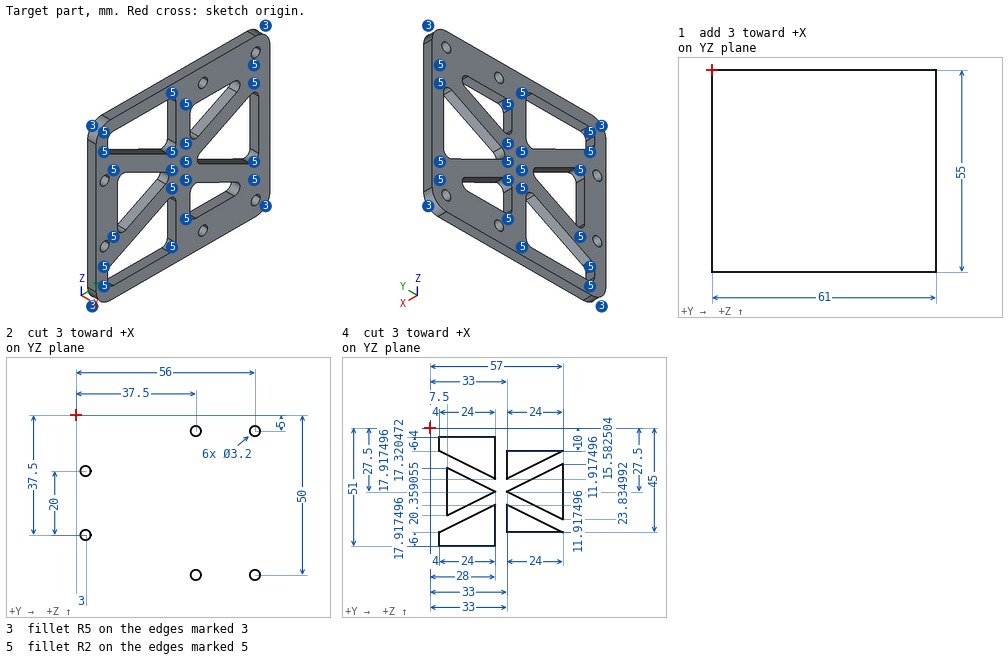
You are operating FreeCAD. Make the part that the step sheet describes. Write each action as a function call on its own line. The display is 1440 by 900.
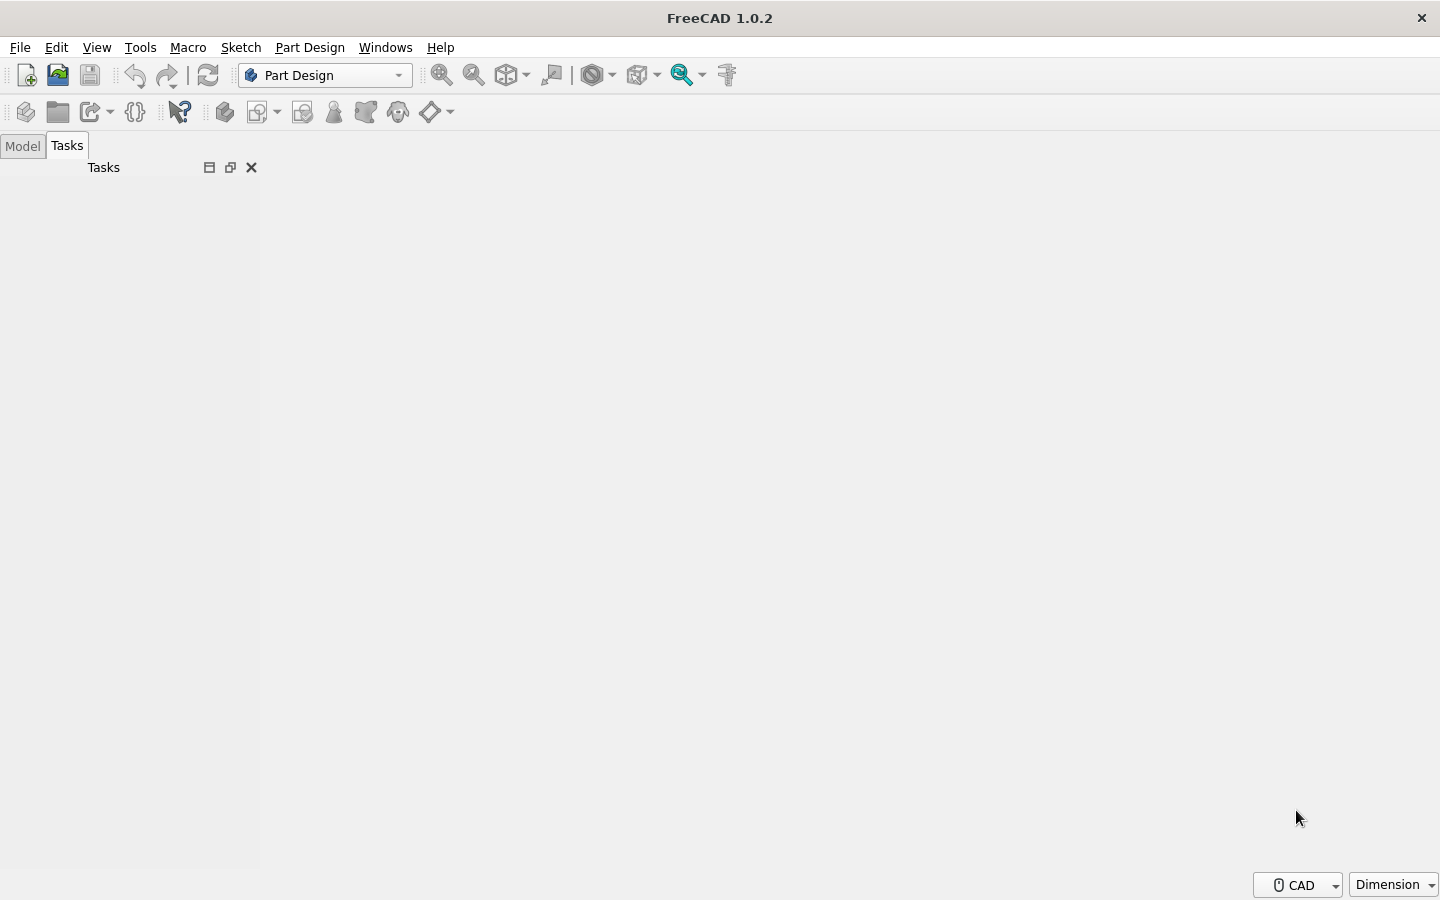
key(ctrl+n)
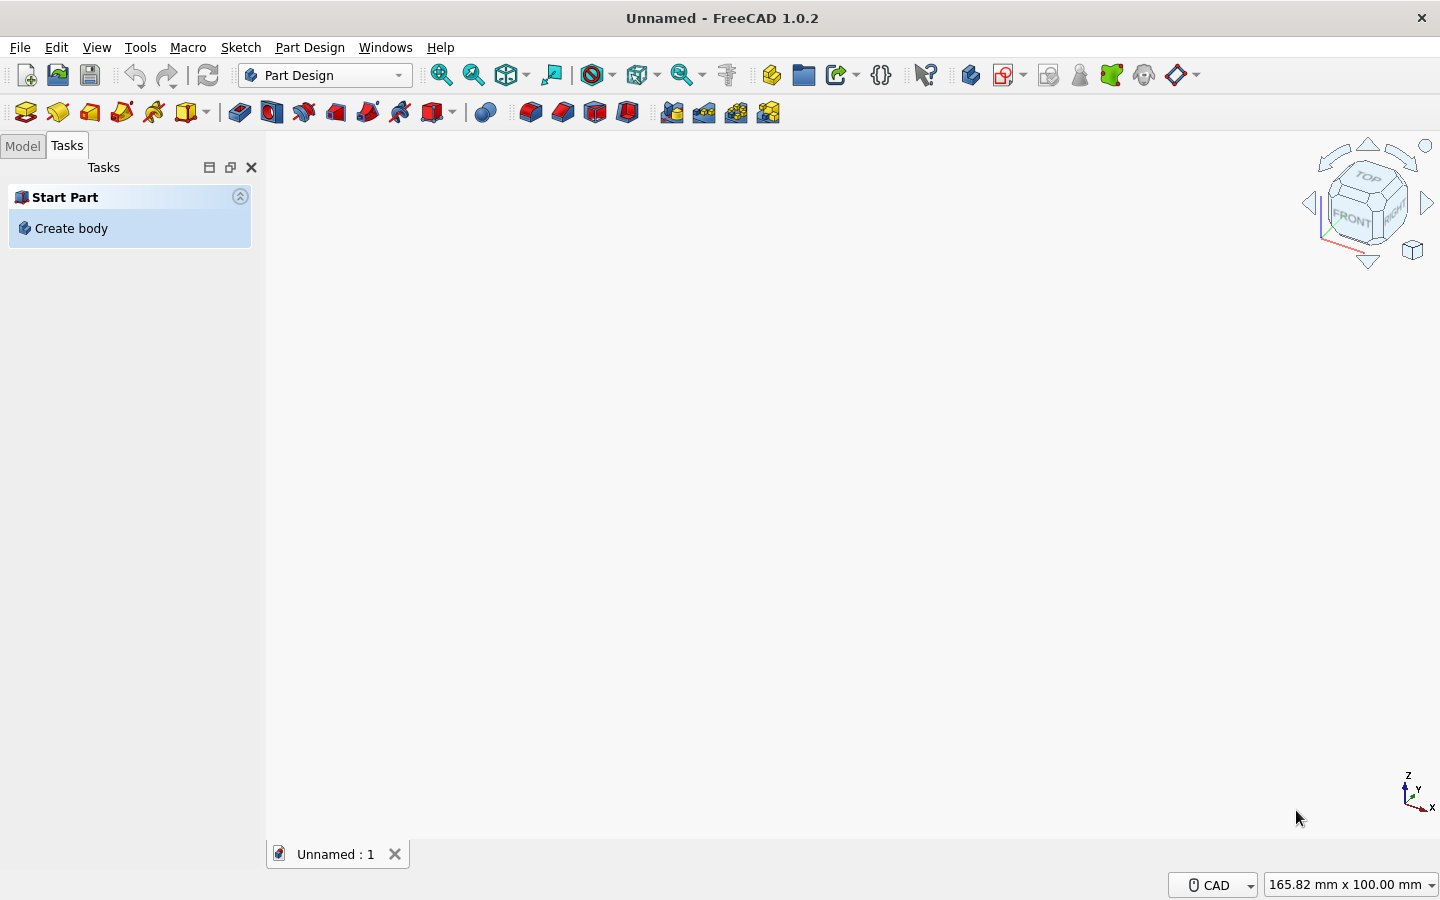
click(1004, 76)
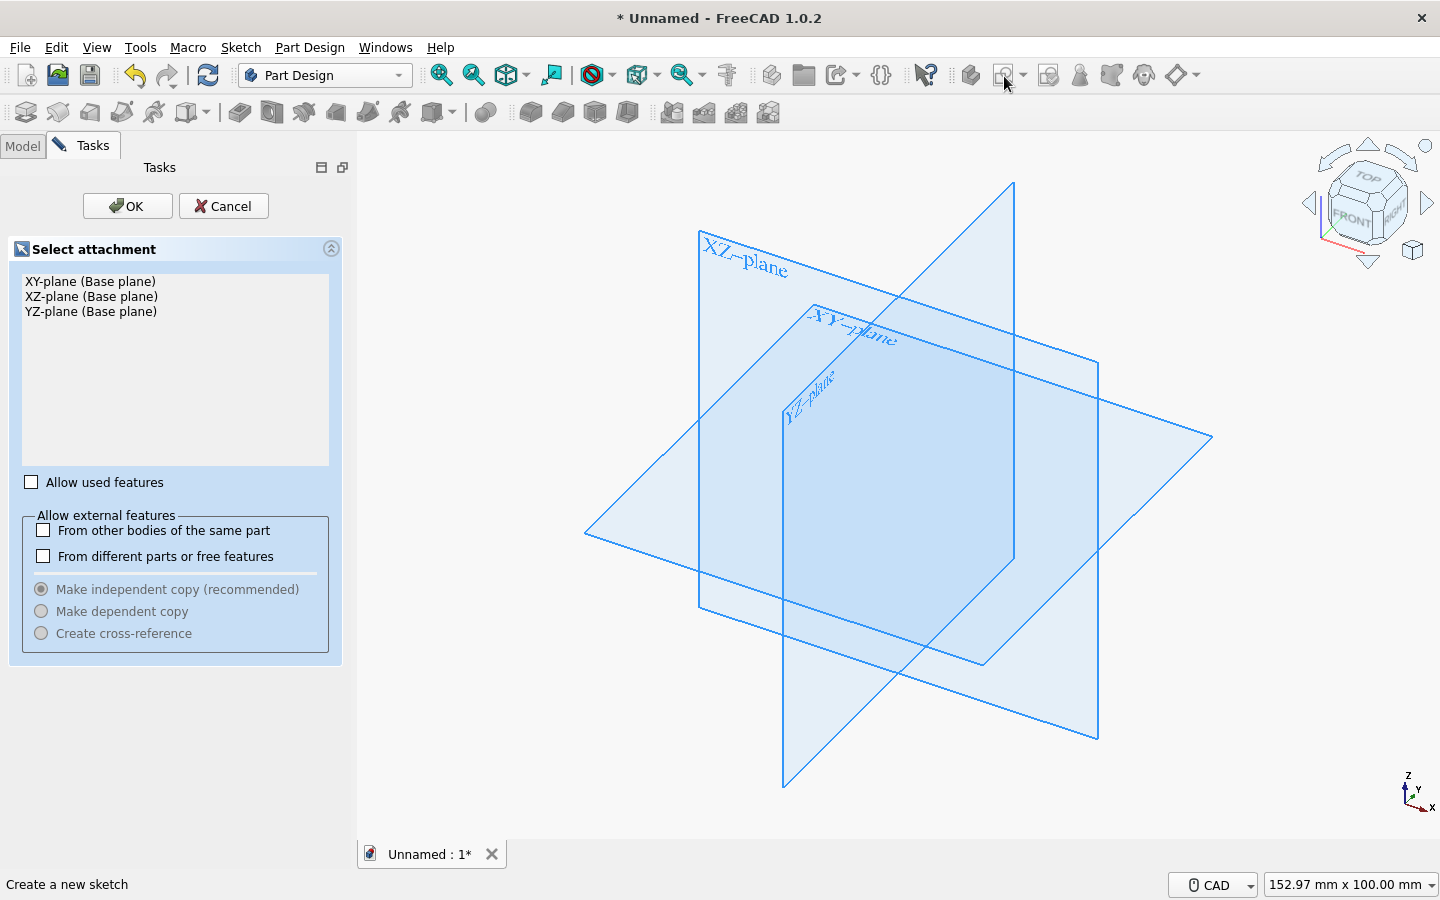
click(82, 312)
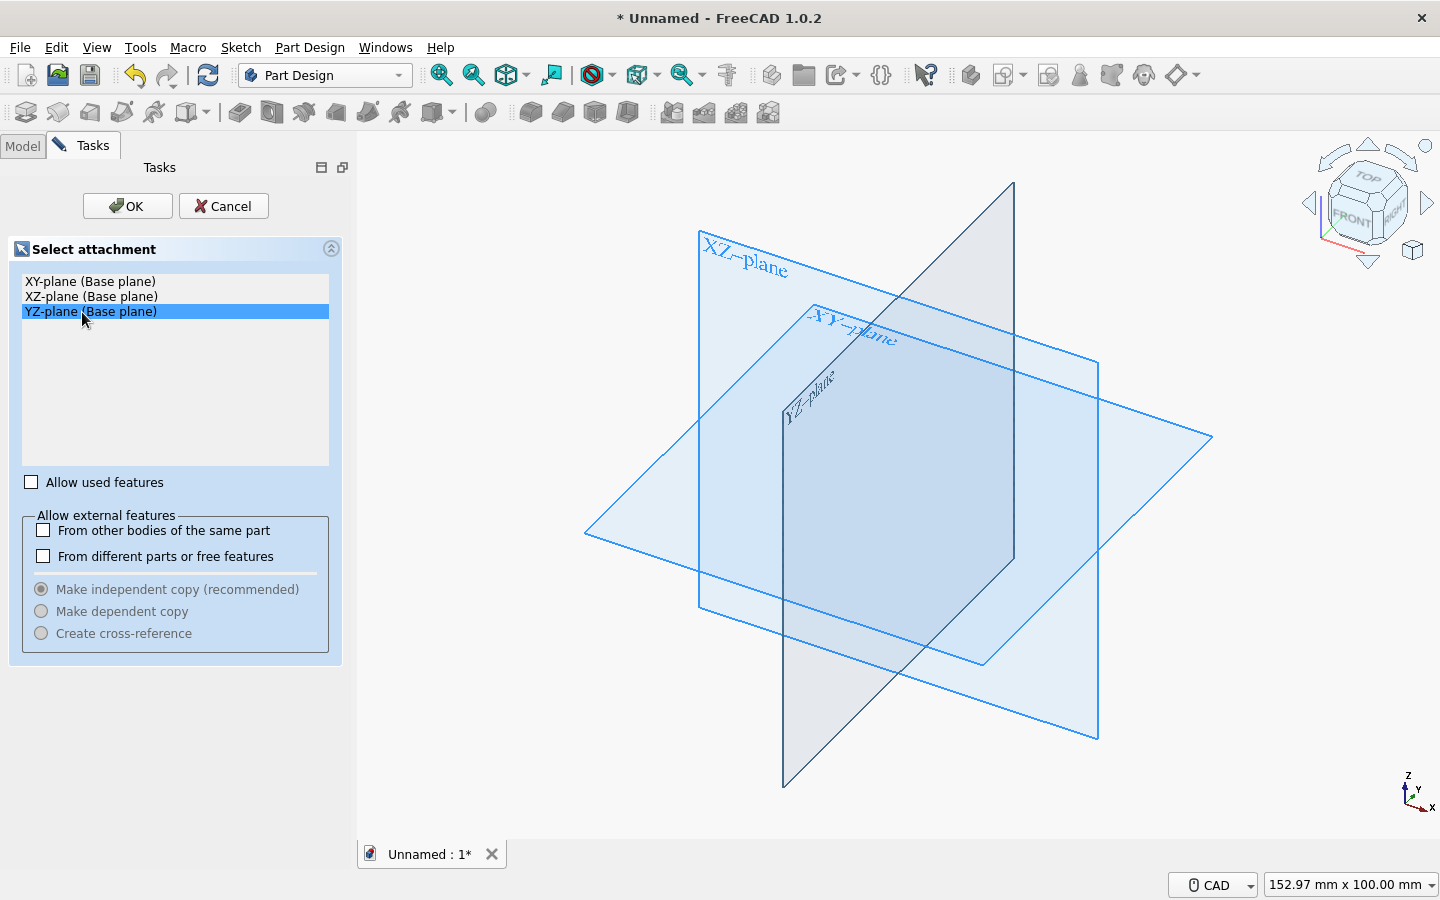
click(128, 206)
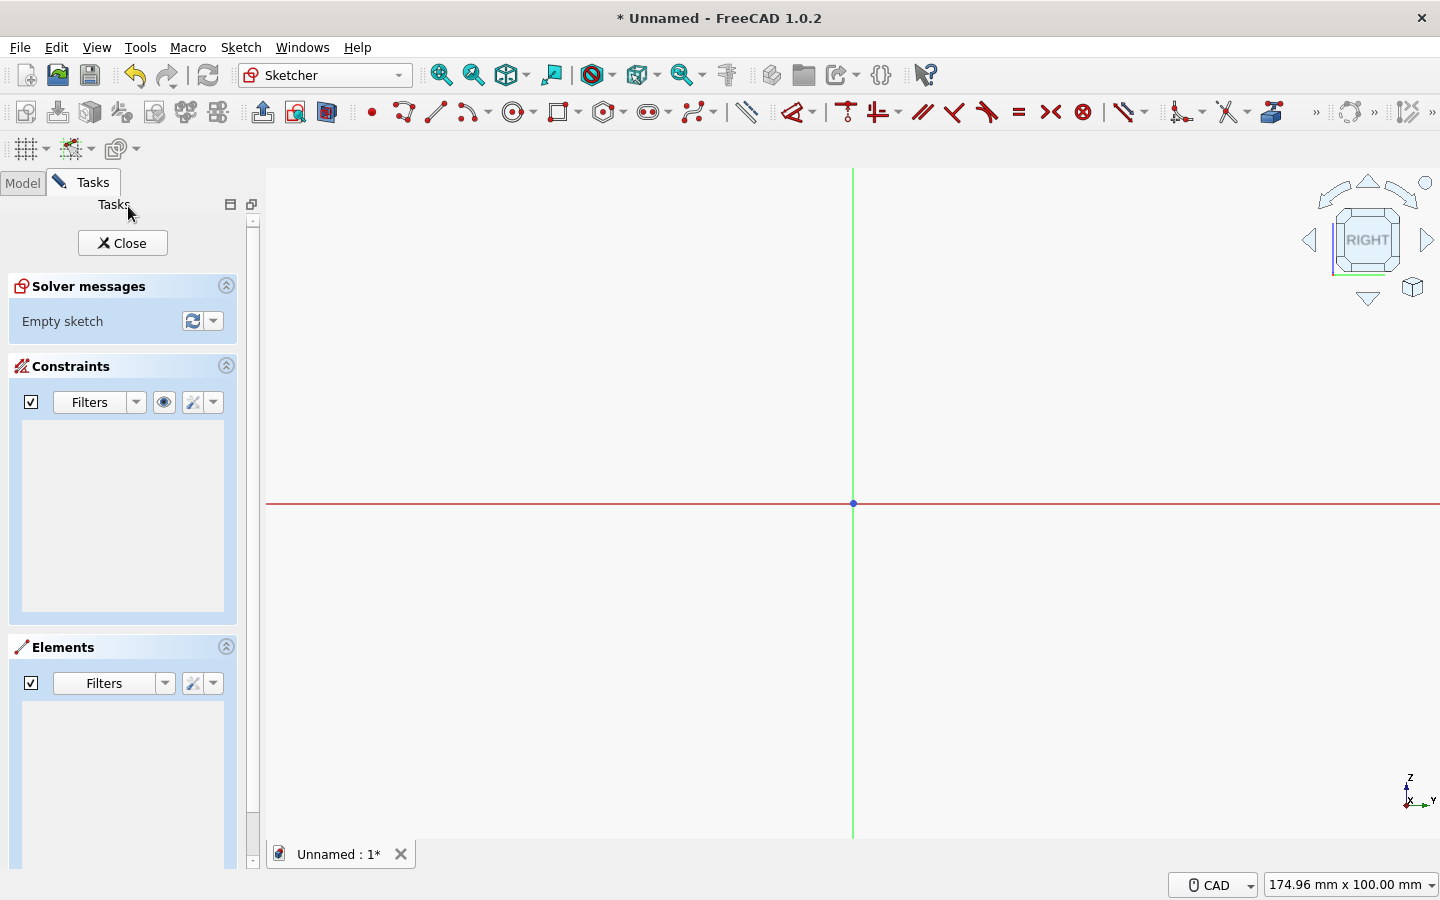
scroll(294, 196, down, 1)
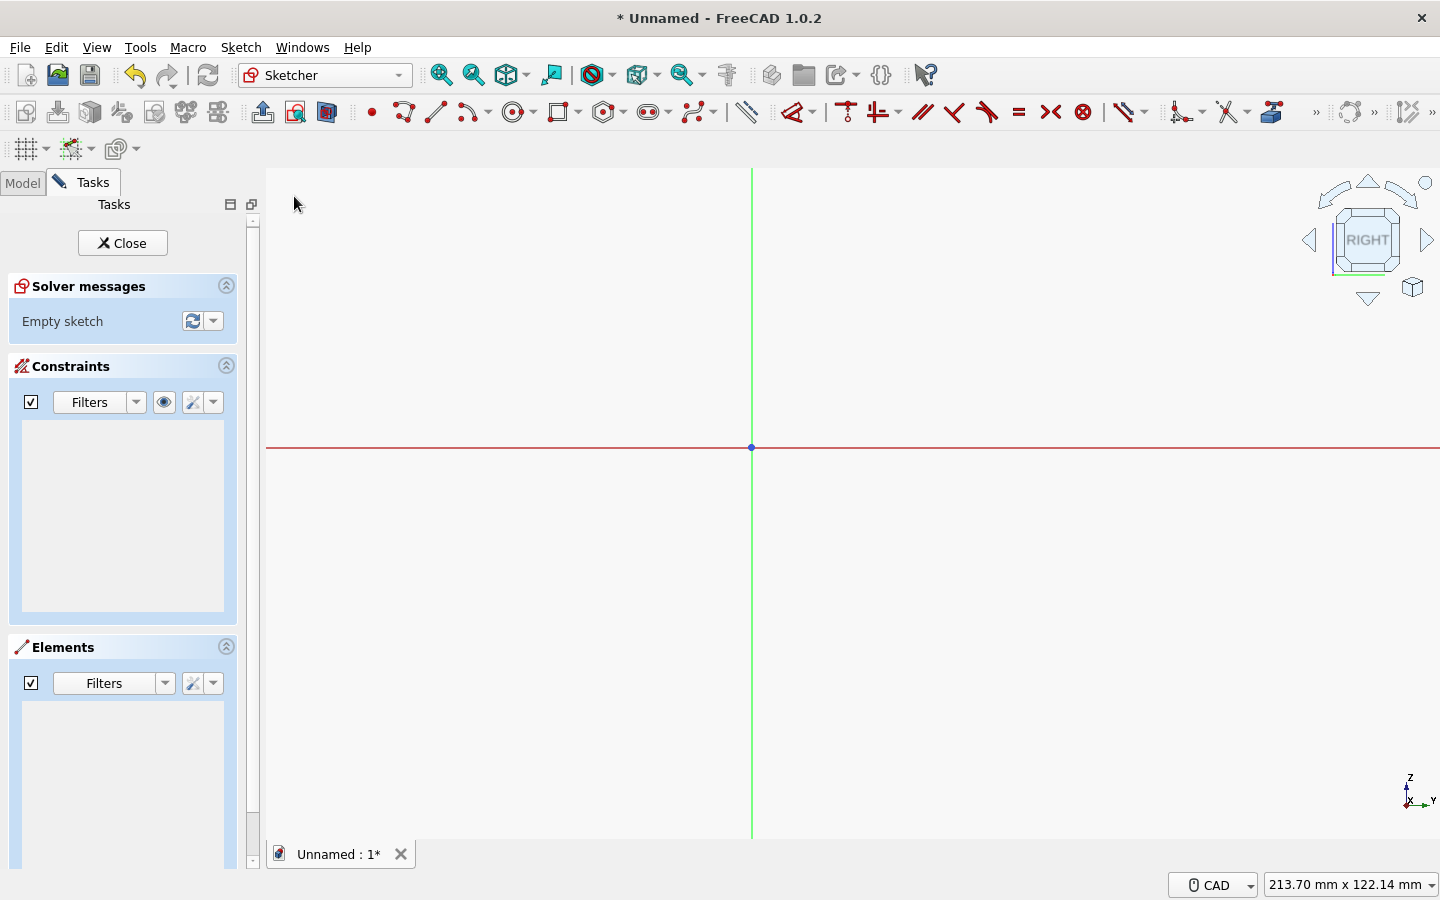
scroll(1193, 793, up, 2)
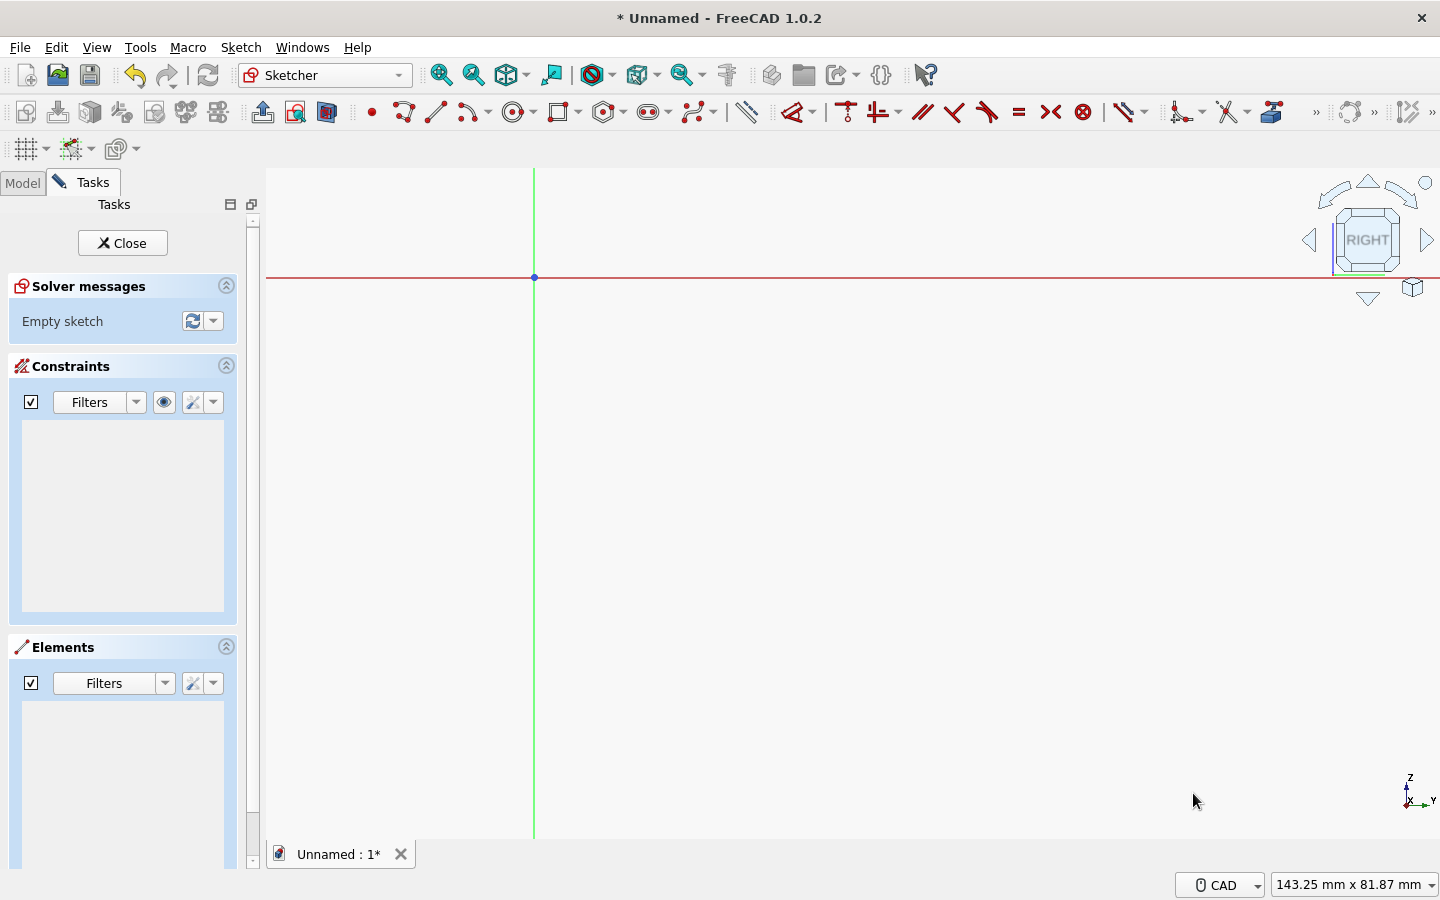
click(558, 112)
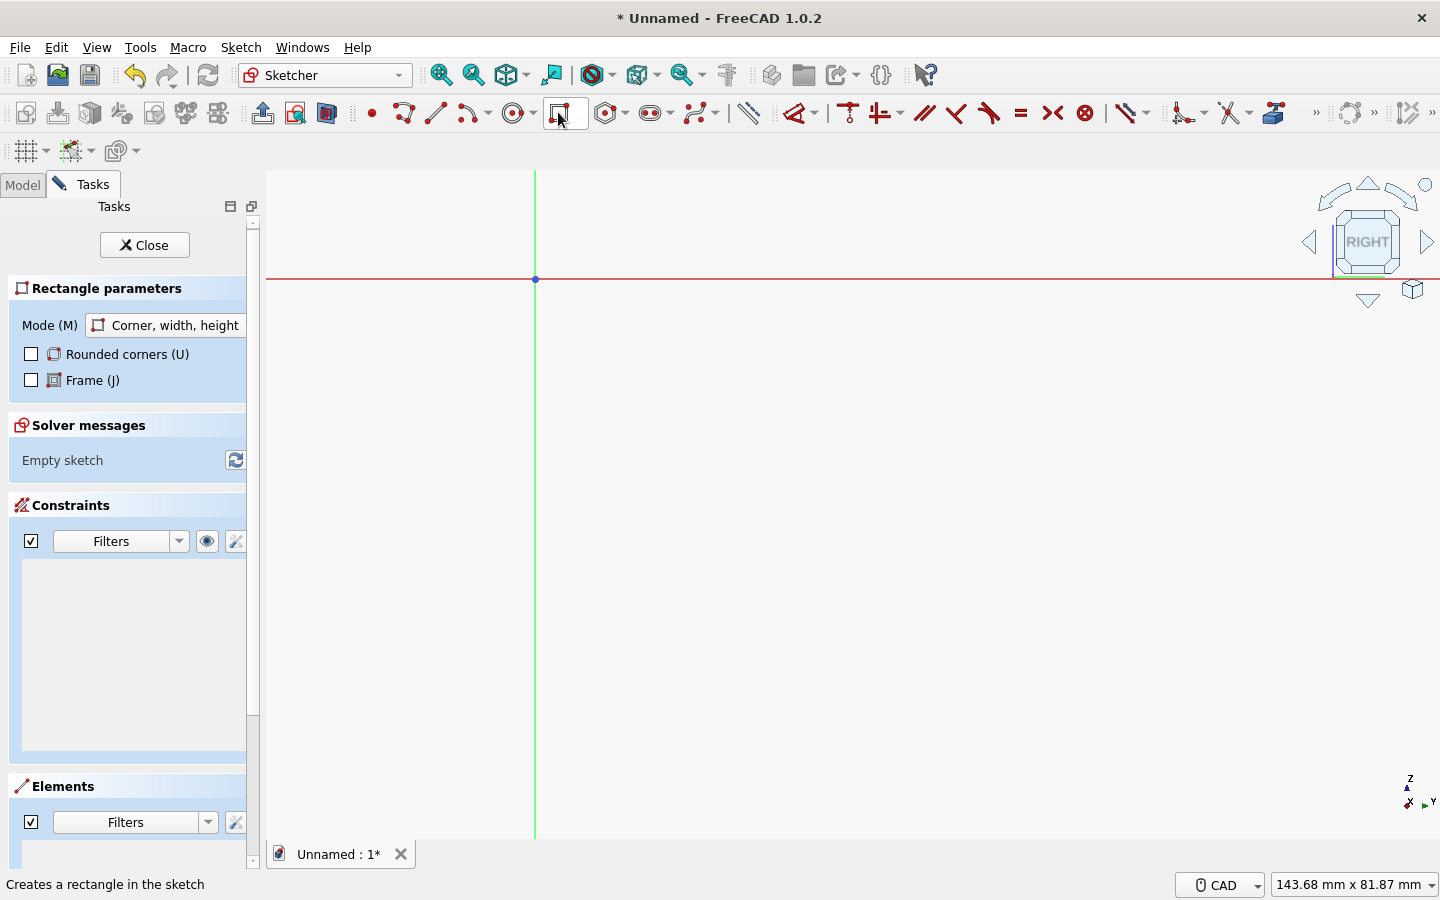
click(535, 279)
move(1034, 729)